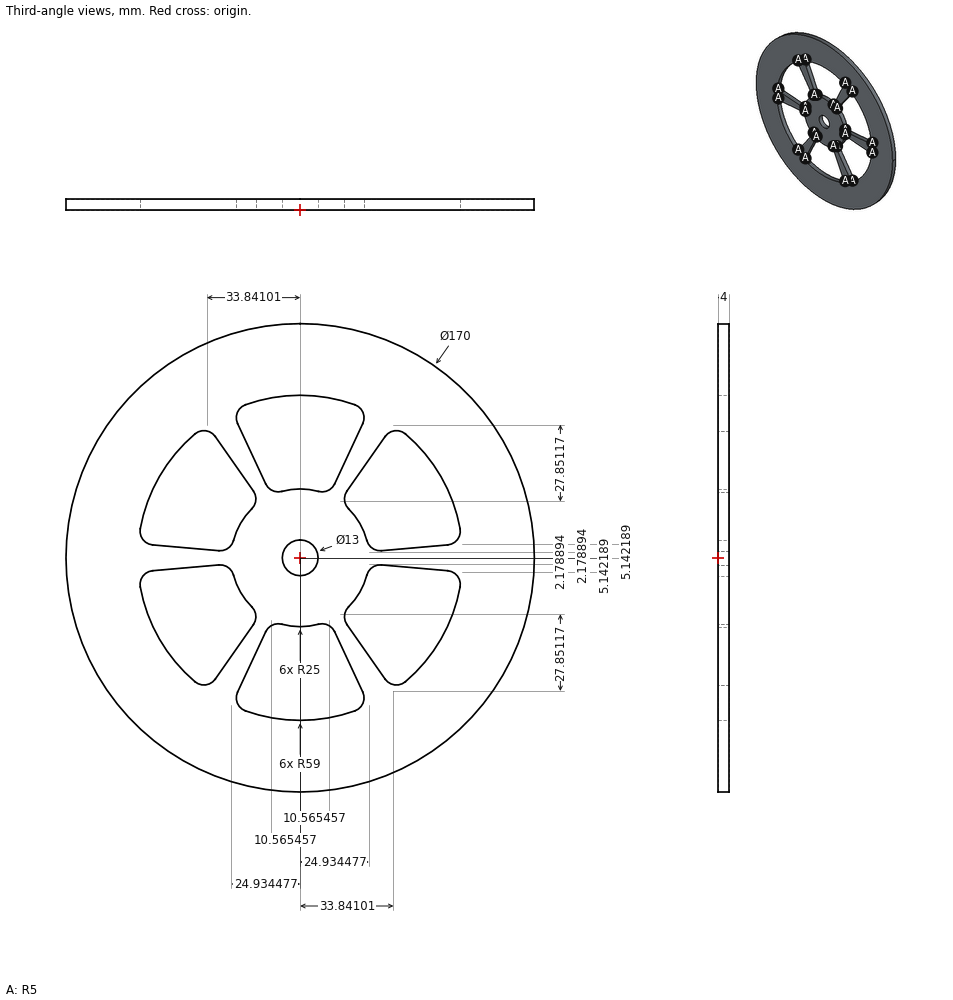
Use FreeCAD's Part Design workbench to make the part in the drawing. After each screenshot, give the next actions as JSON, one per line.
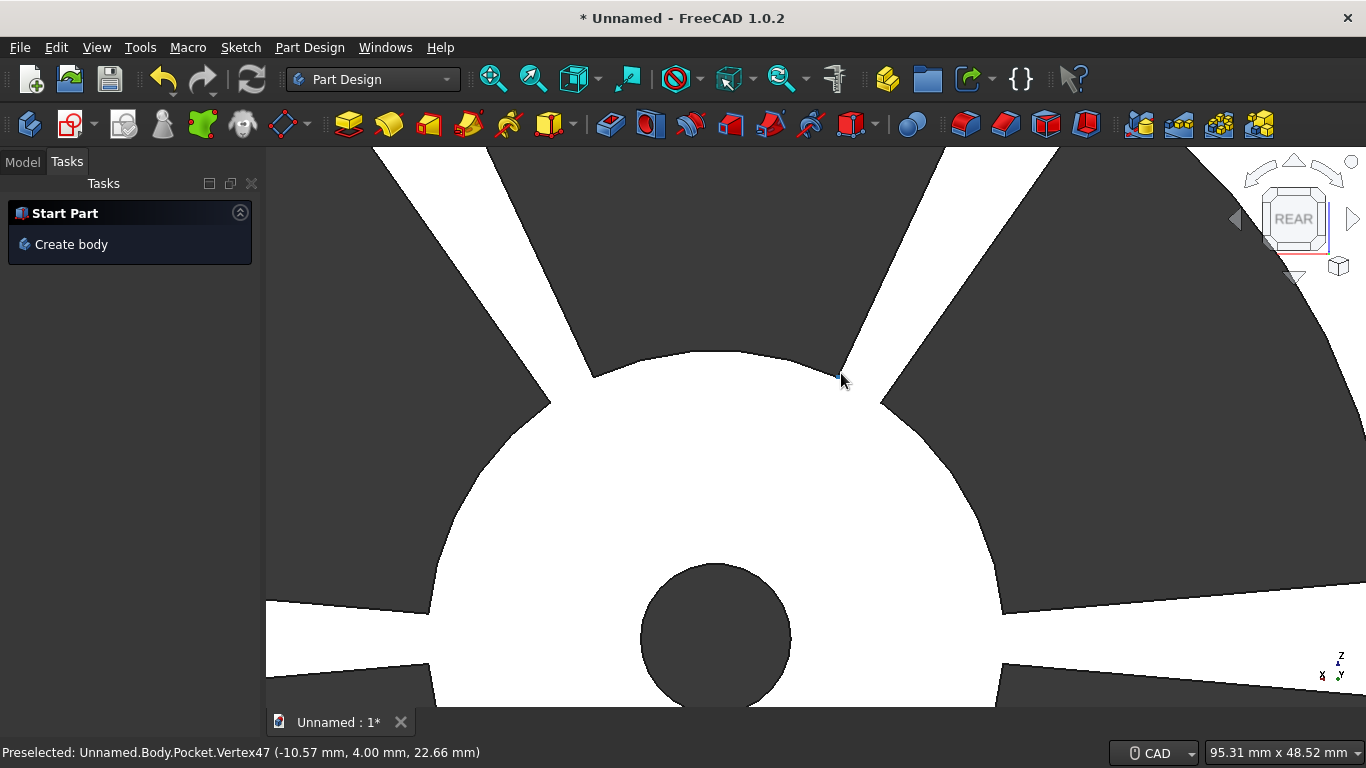
{"action": "left_click", "coordinate": [494, 80]}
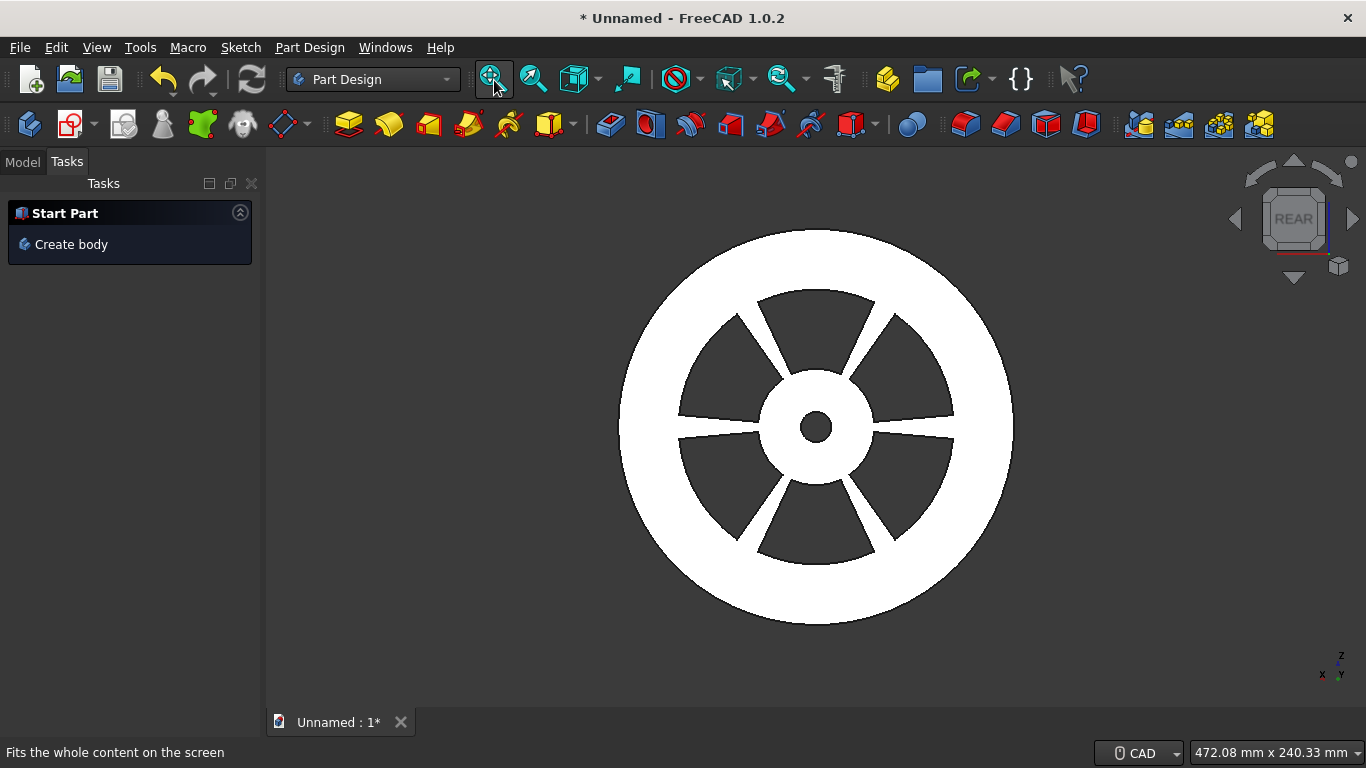
{"action": "key", "text": "0"}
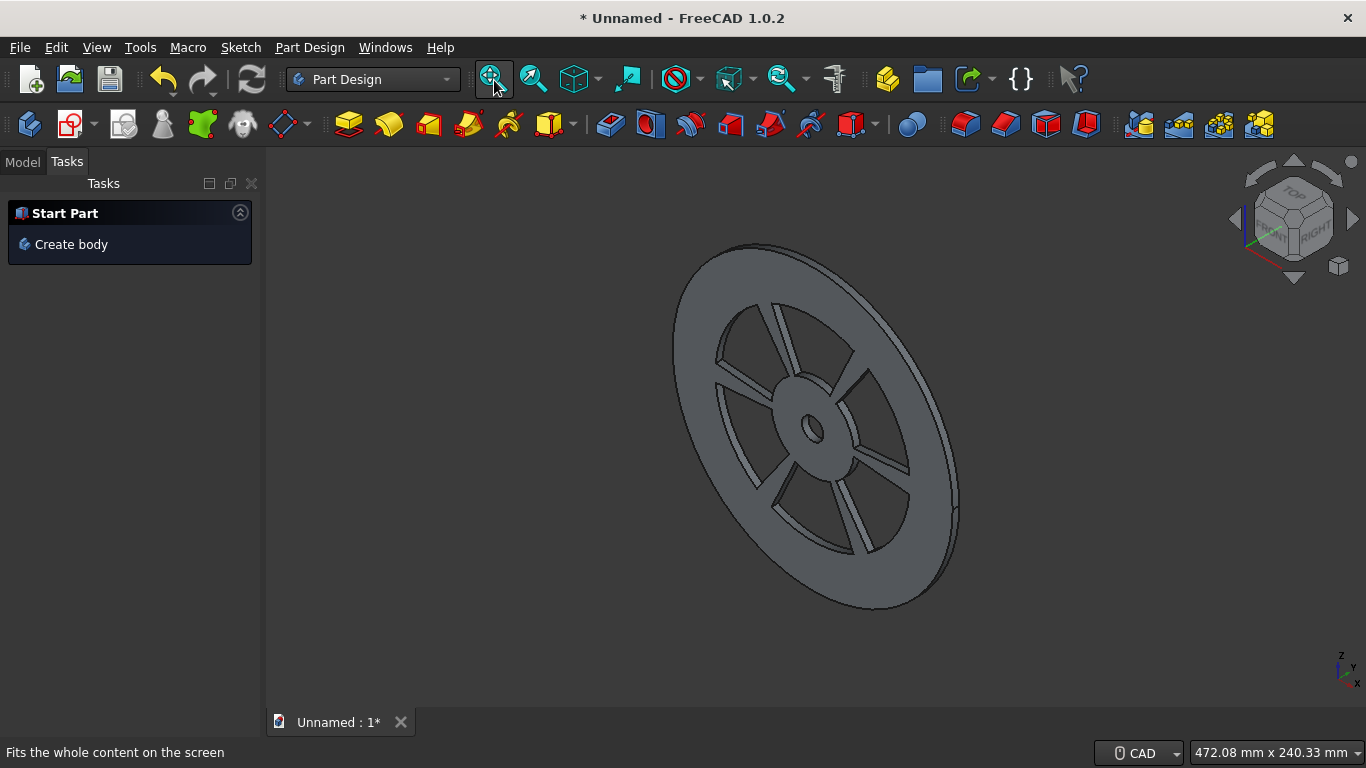
{"action": "scroll", "coordinate": [798, 373], "scroll_direction": "up", "scroll_amount": 8}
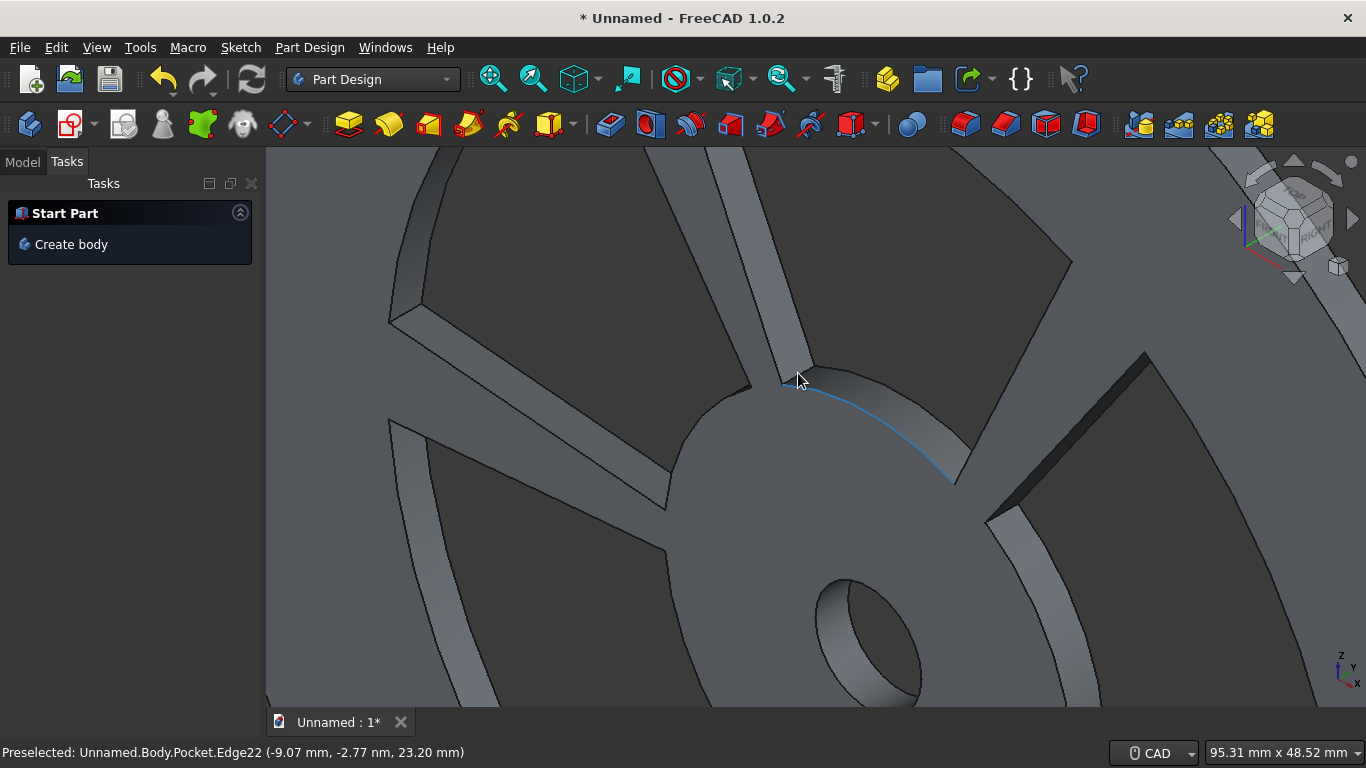
{"action": "left_click", "coordinate": [494, 80]}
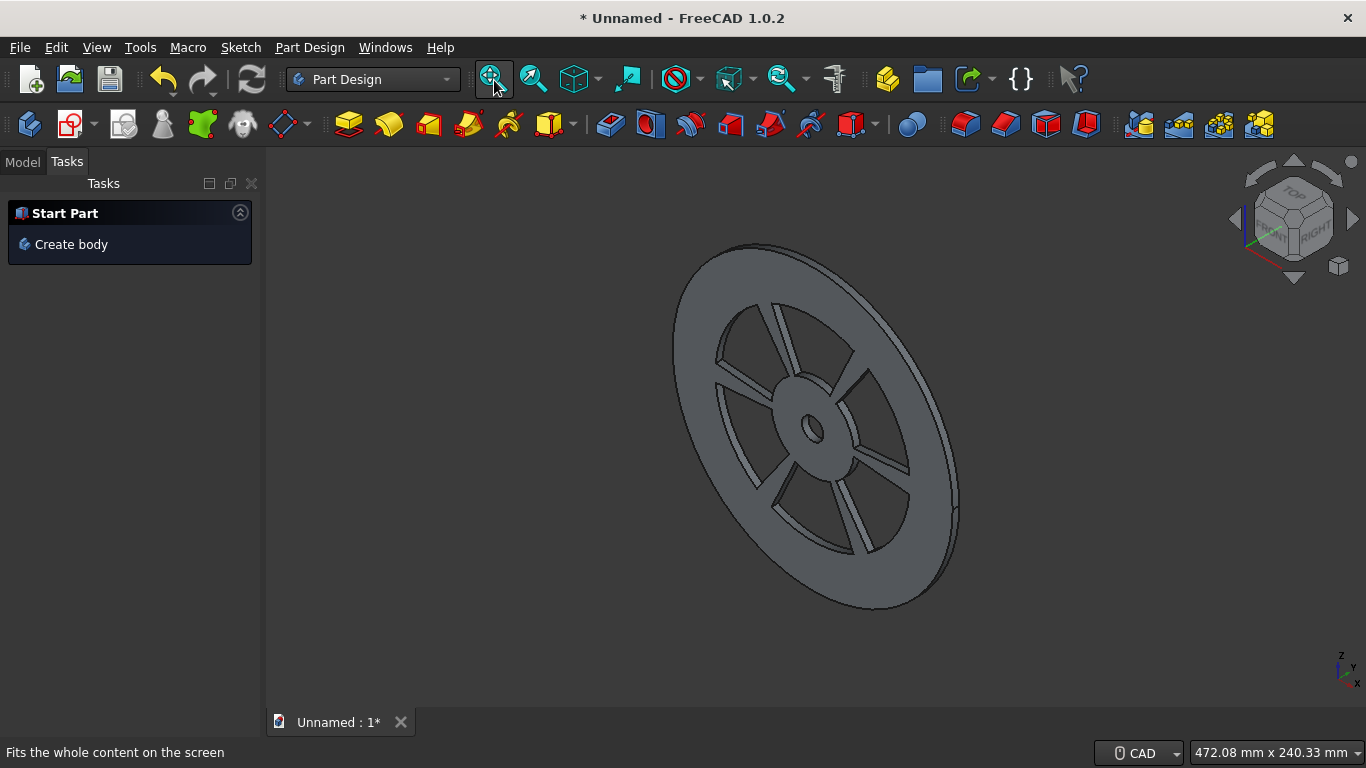
{"action": "key", "text": "2"}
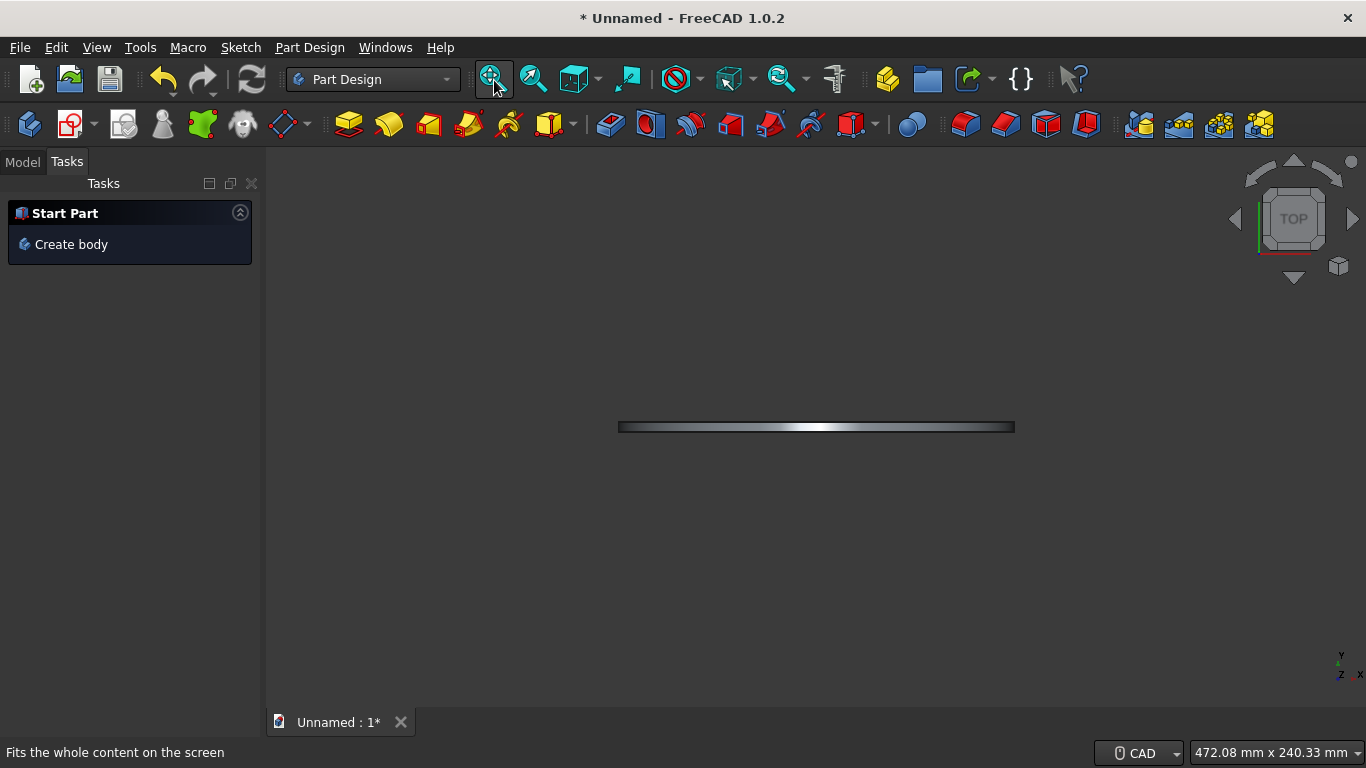
{"action": "left_click", "coordinate": [494, 80]}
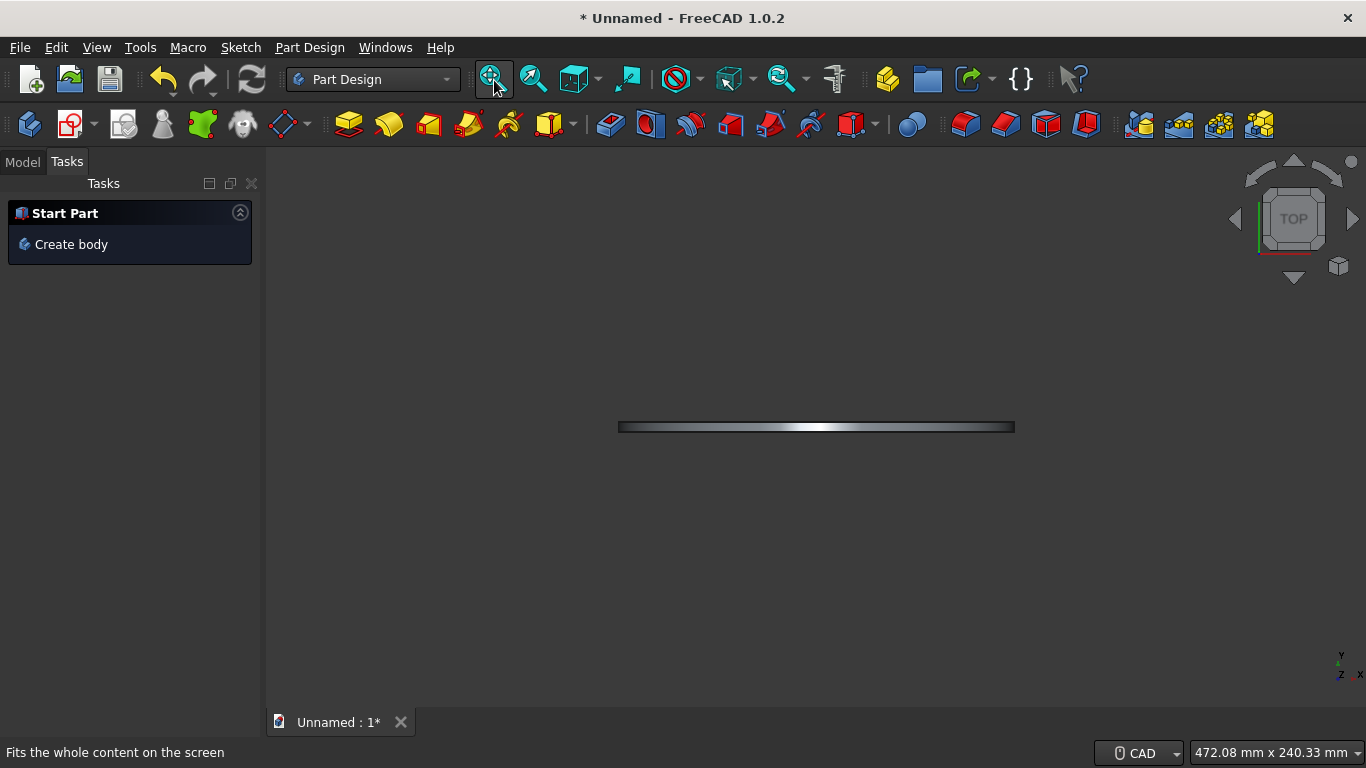
{"action": "scroll", "coordinate": [791, 426], "scroll_direction": "up", "scroll_amount": 8}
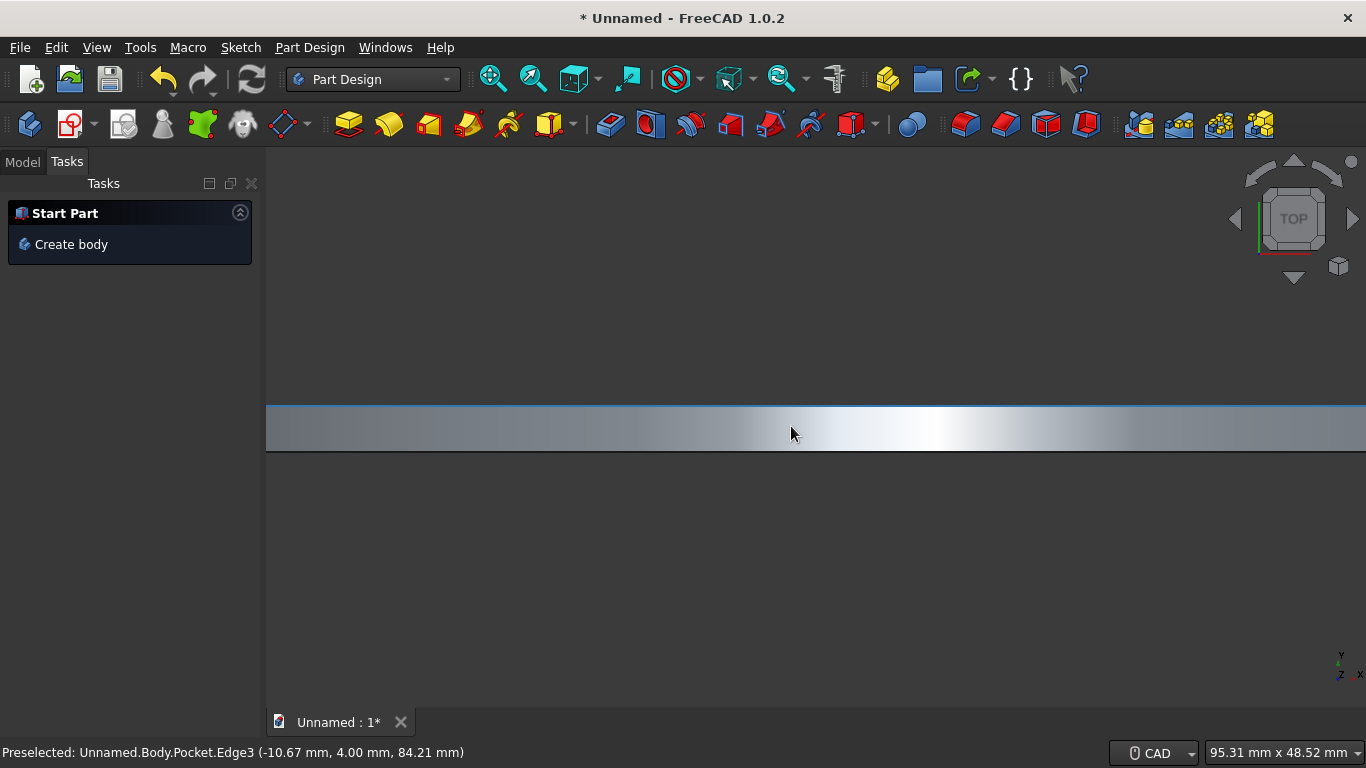
{"action": "left_click", "coordinate": [494, 80]}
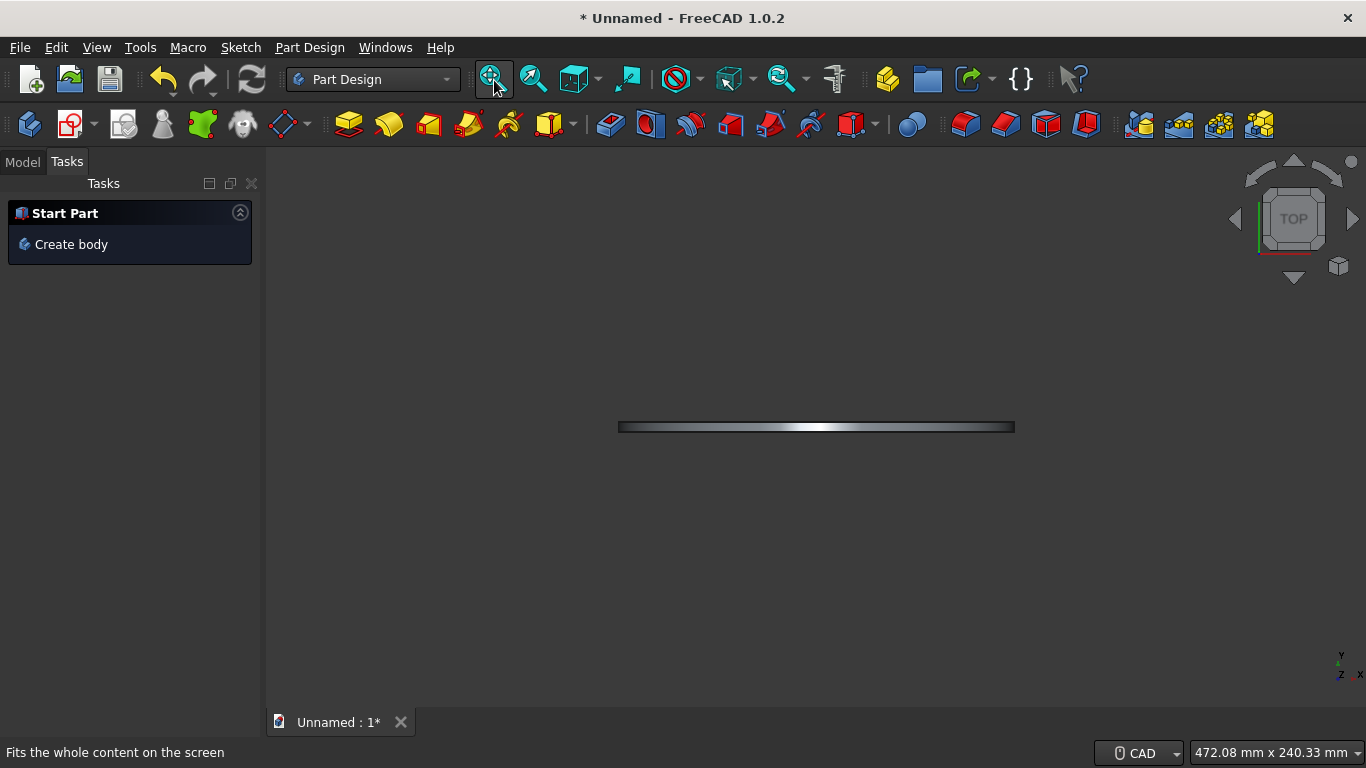
{"action": "key", "text": "1"}